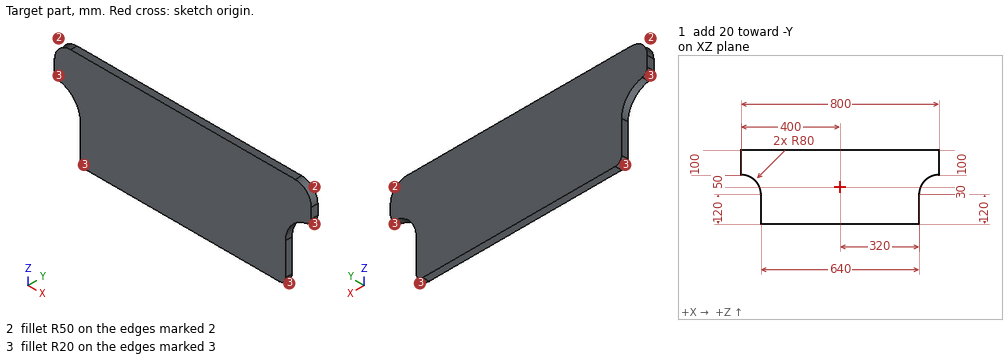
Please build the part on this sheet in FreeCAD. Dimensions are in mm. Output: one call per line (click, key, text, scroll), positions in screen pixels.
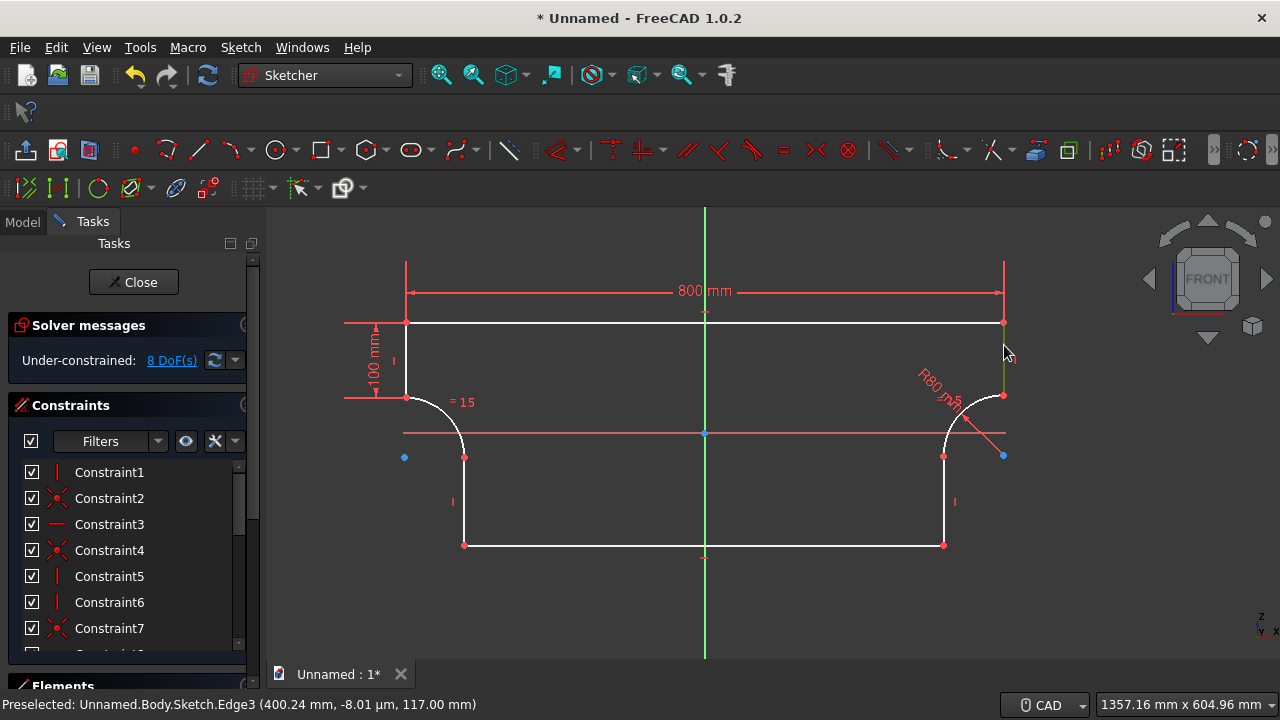
click(580, 150)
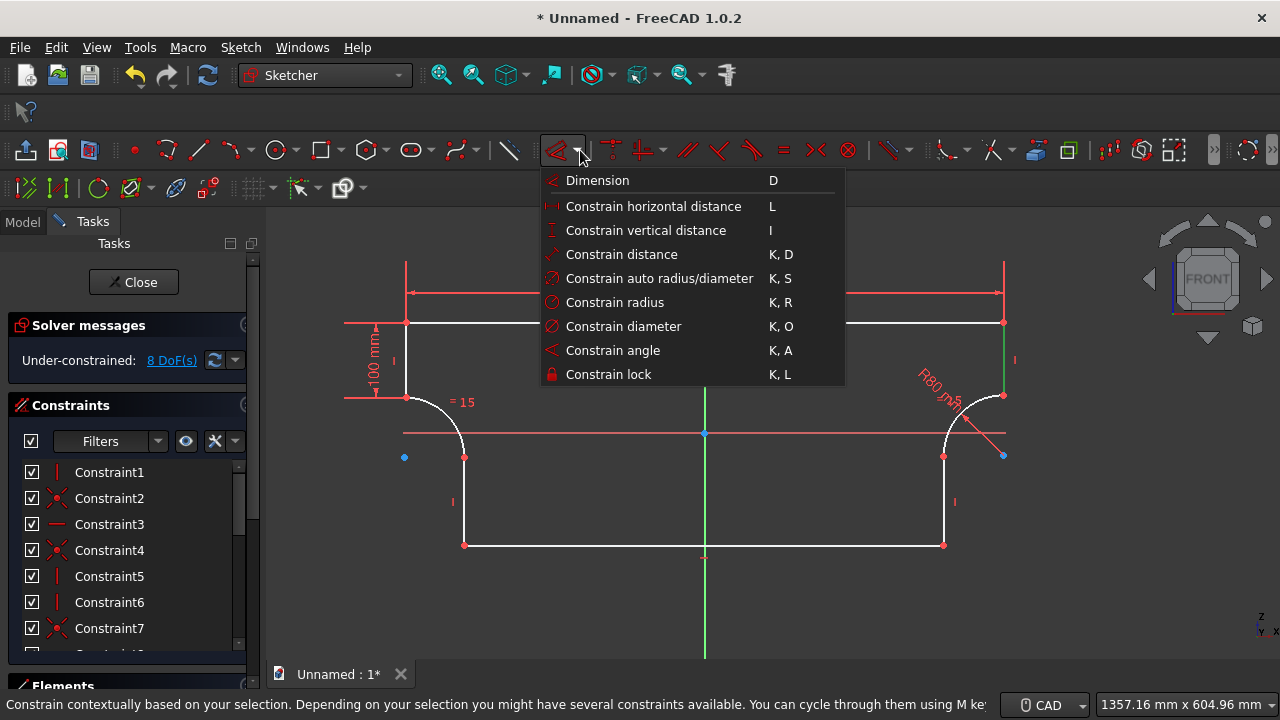
click(693, 230)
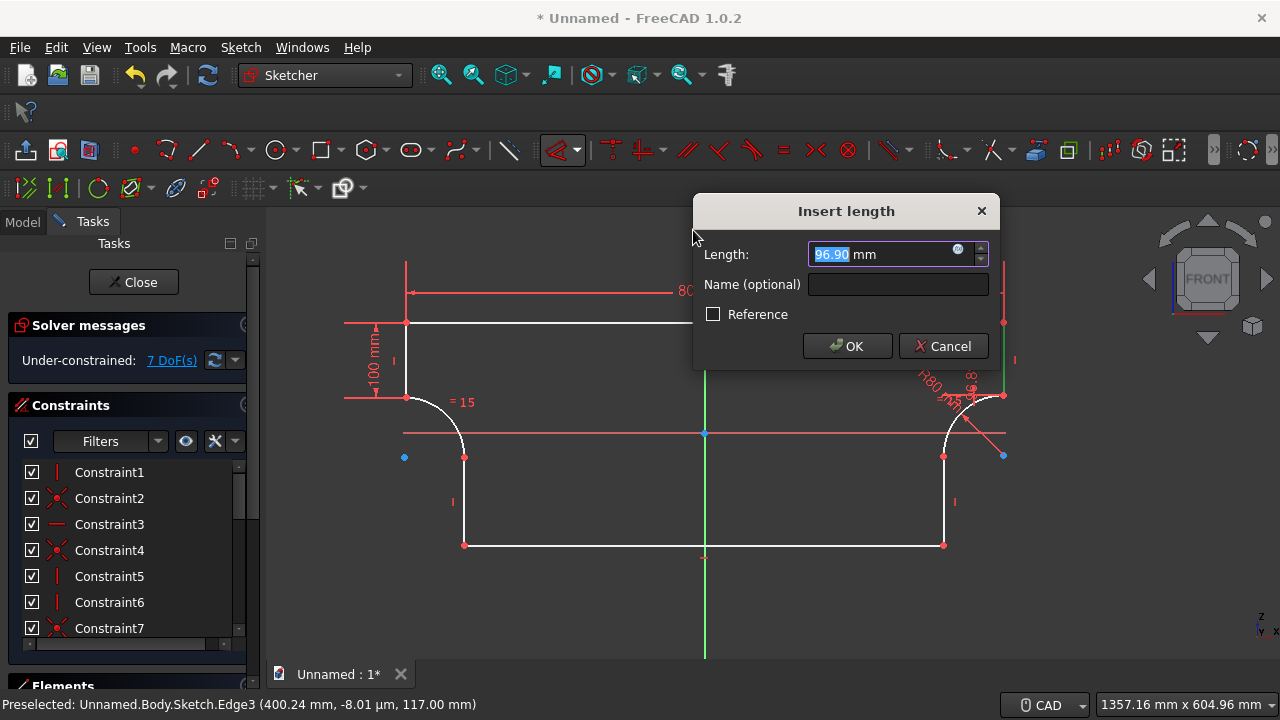
text(100)
key(Return)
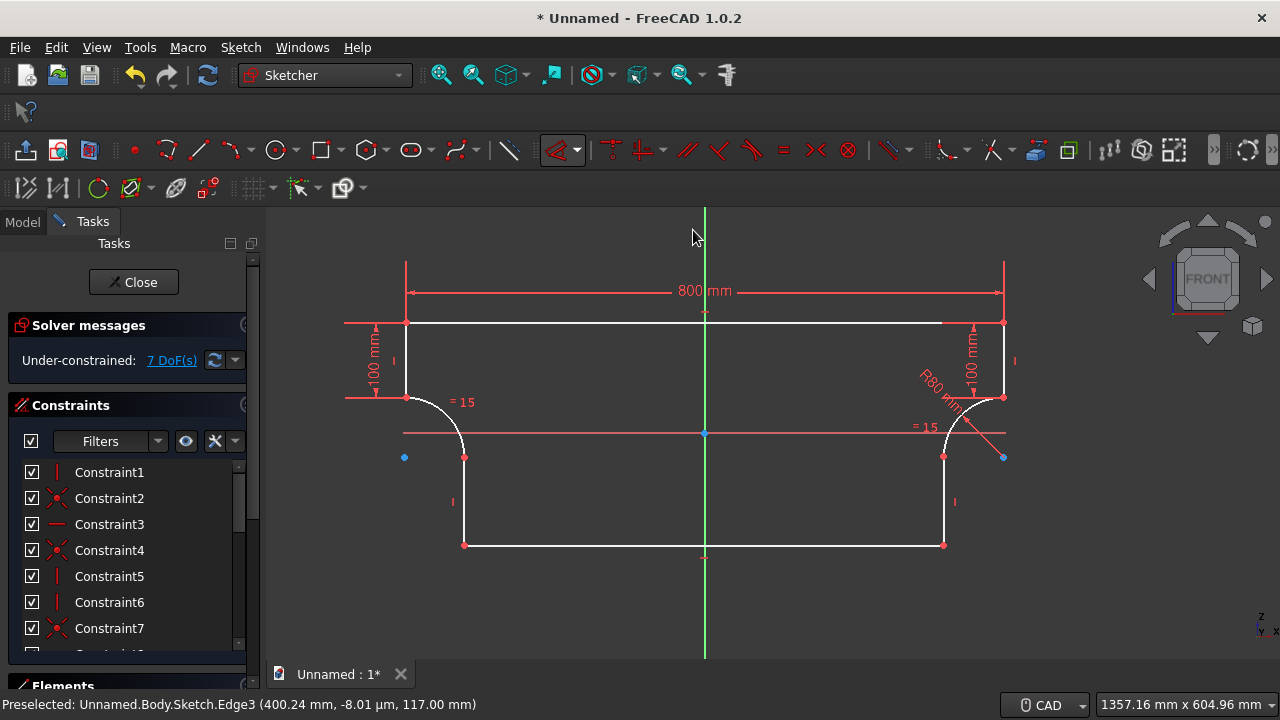
click(944, 484)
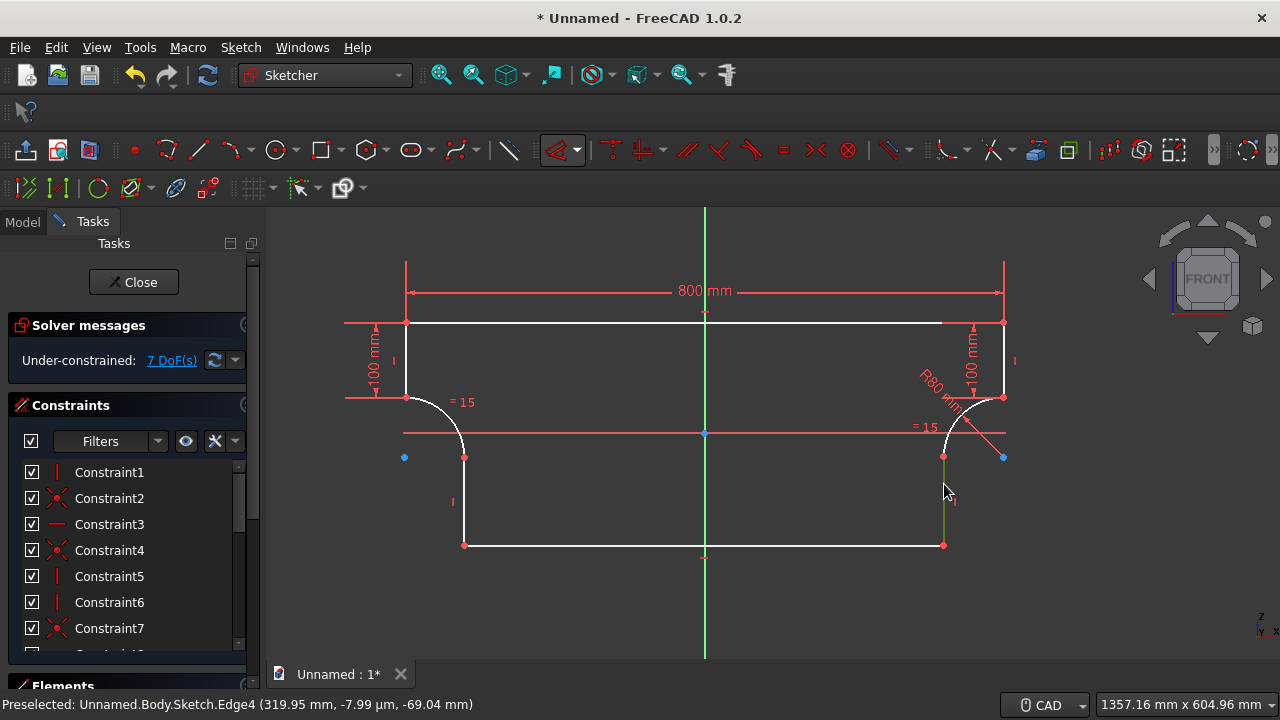
key(i)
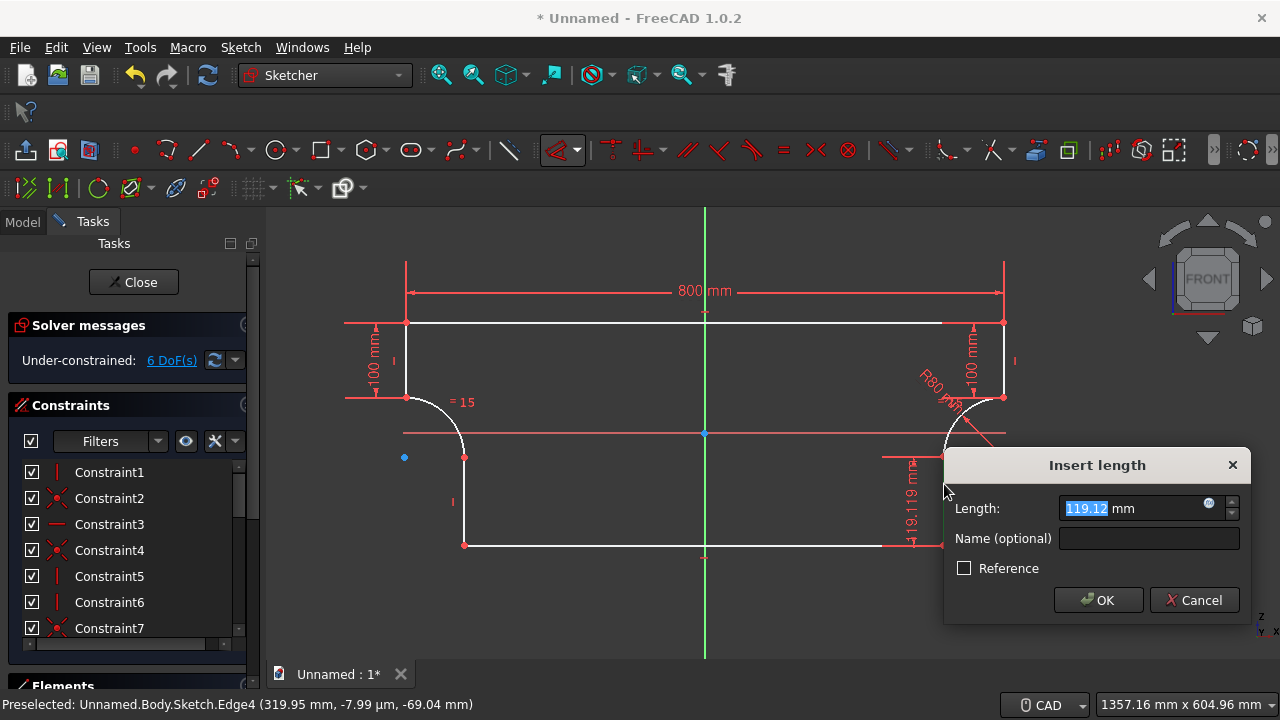
text(120)
key(Return)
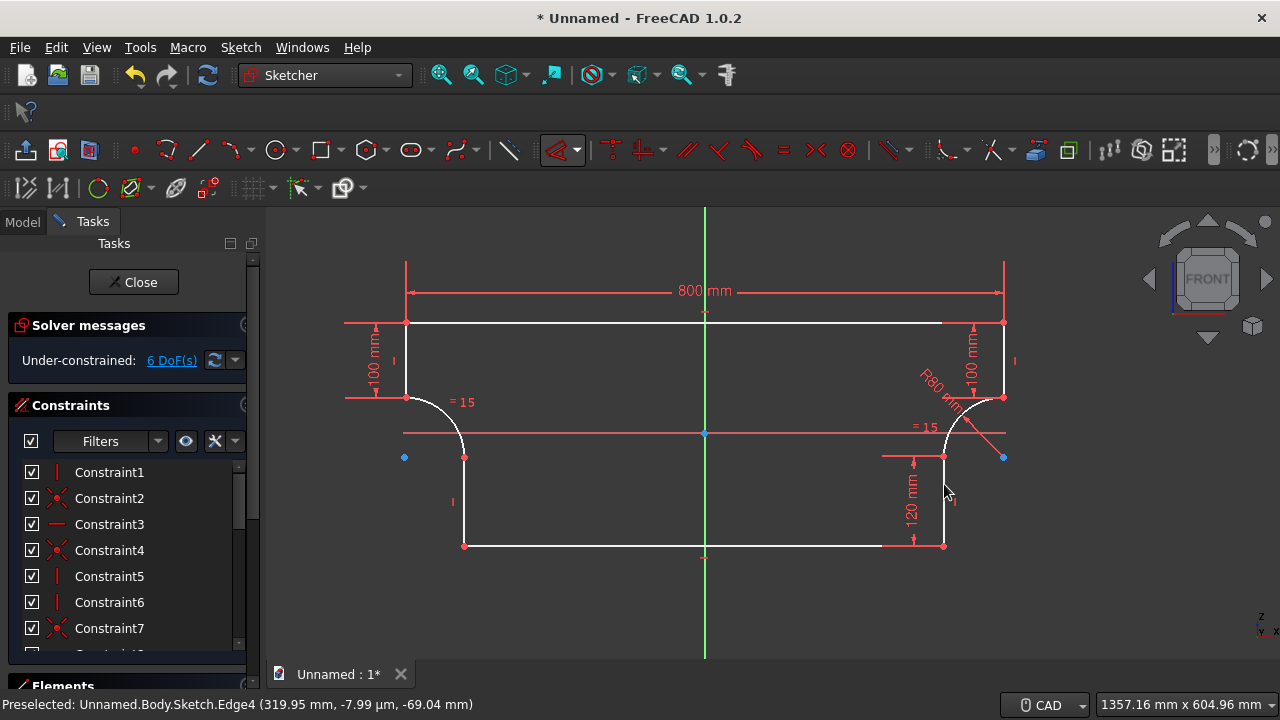
click(800, 546)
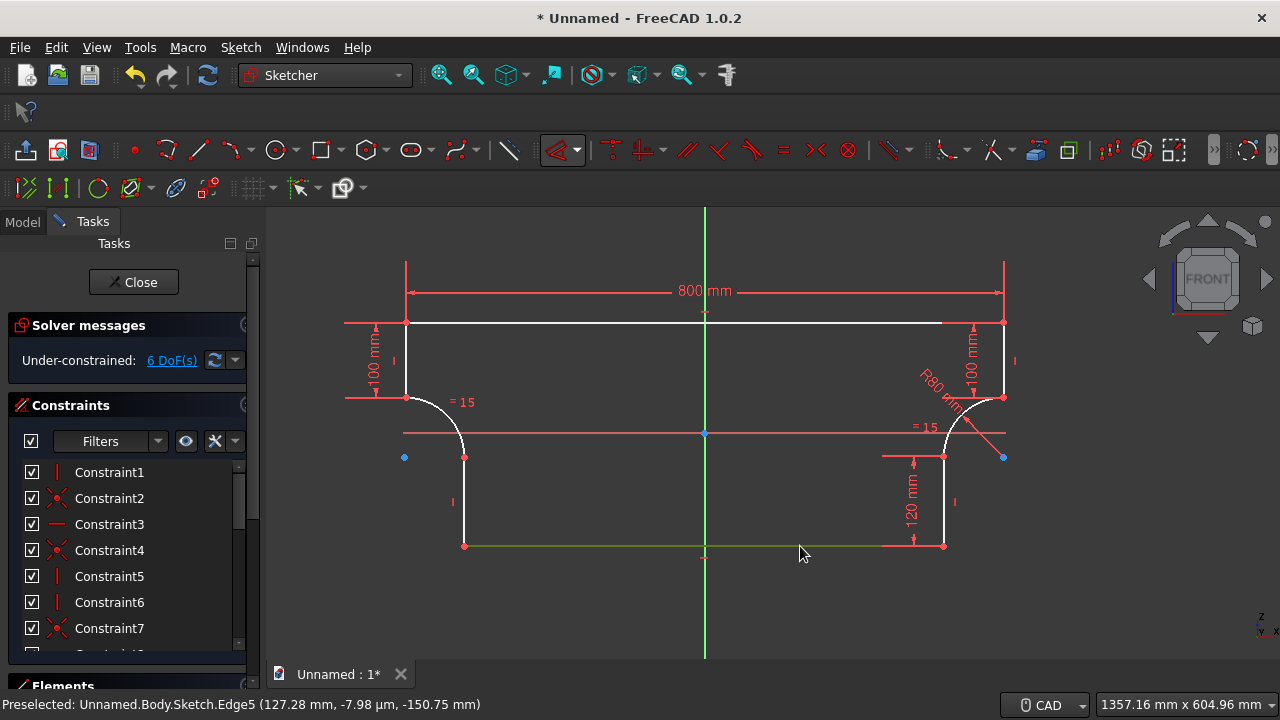
key(l)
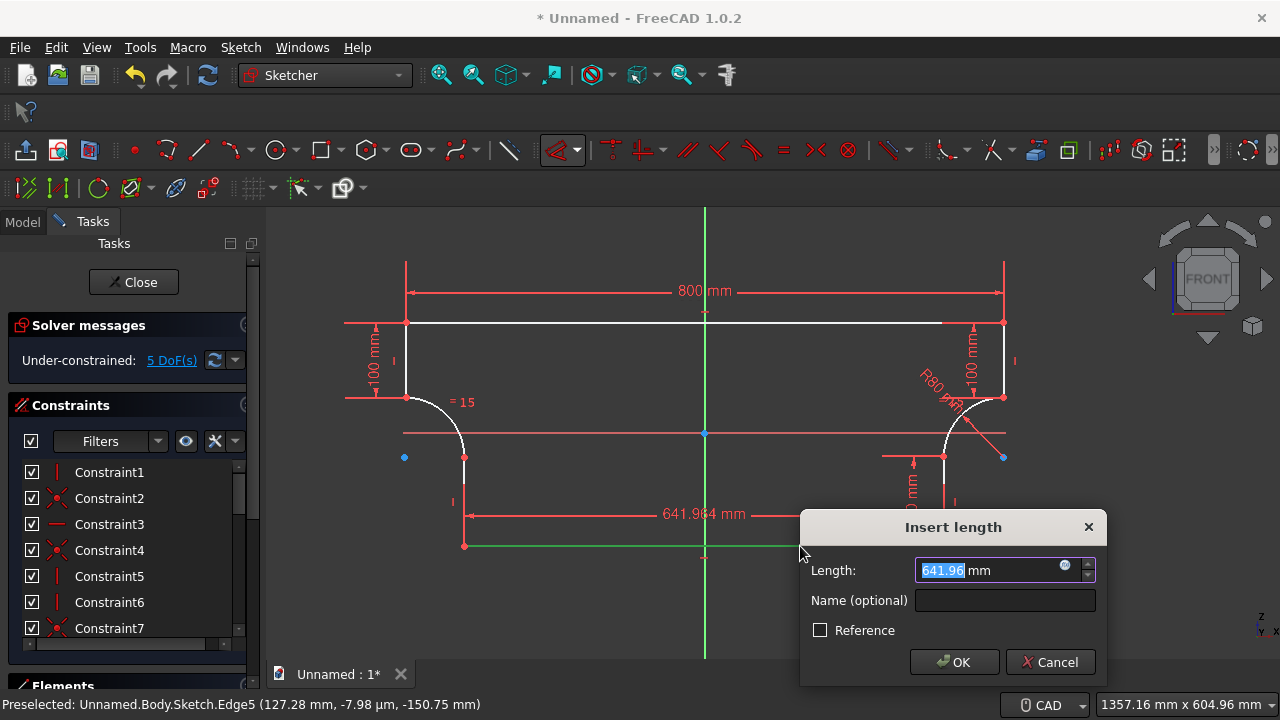
text(640)
key(Return)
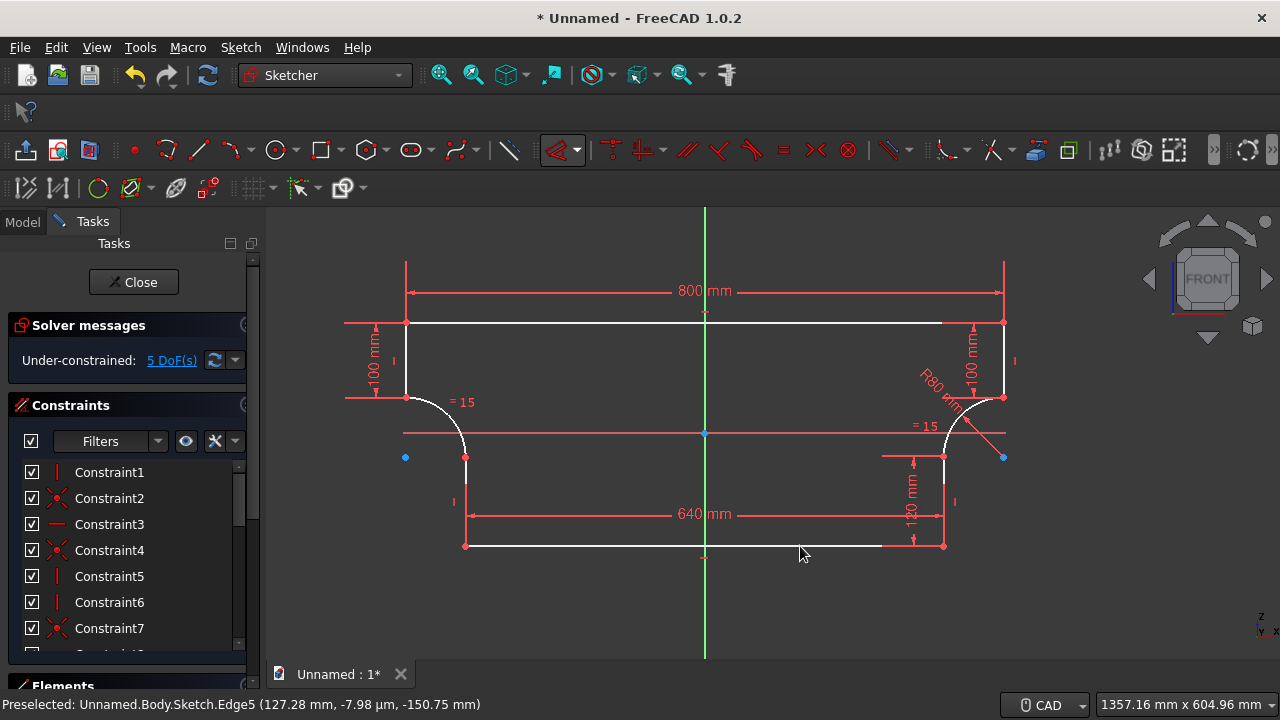
click(466, 519)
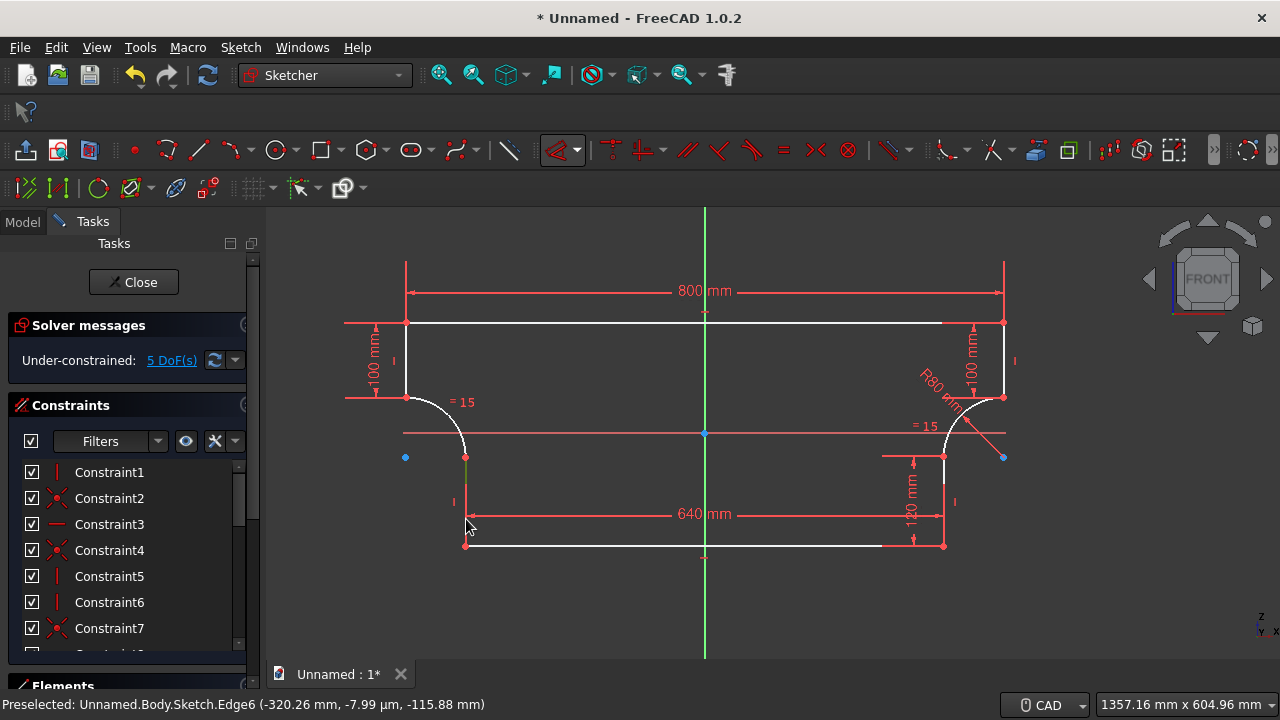
key(i)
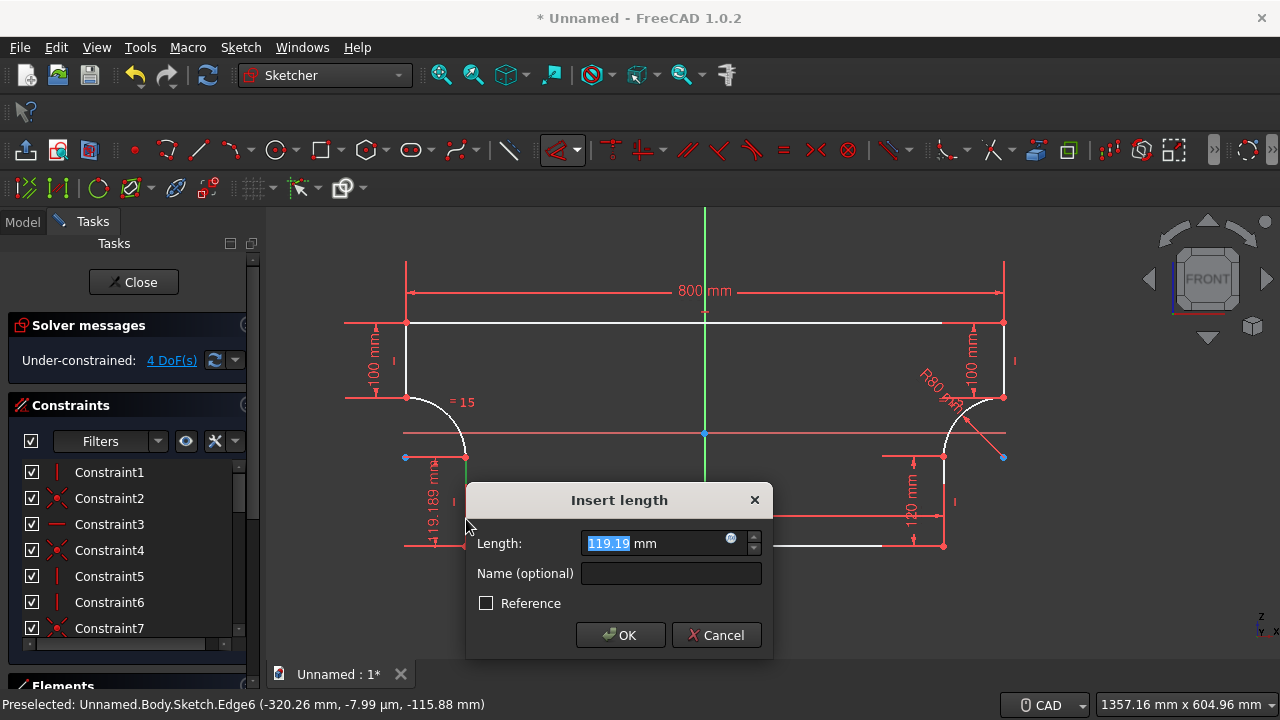
text(120)
key(Return)